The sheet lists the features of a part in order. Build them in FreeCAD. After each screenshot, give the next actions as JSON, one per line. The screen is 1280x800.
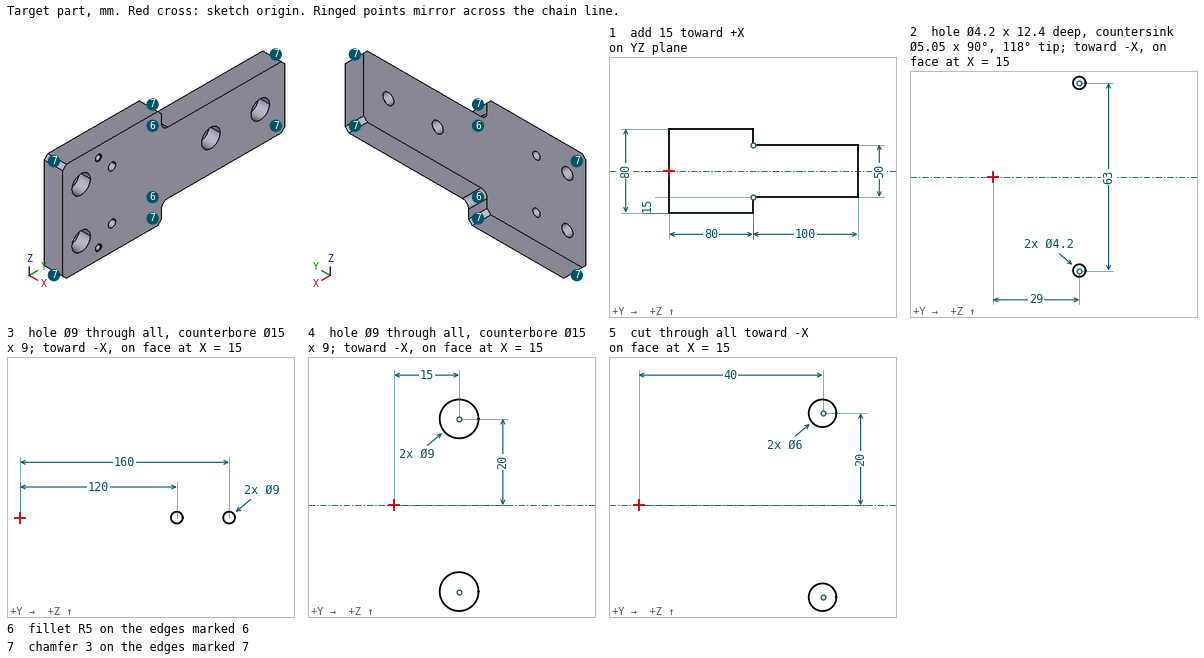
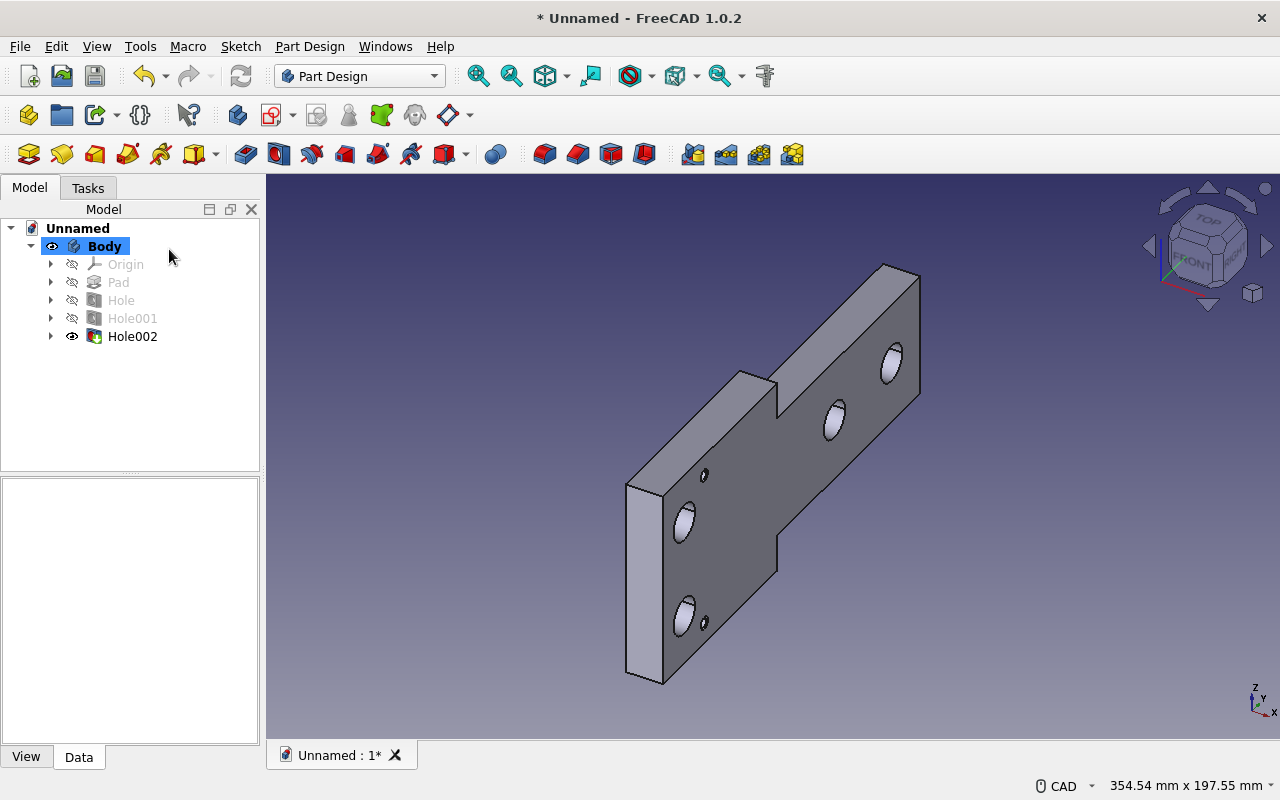
{"action": "left_click", "coordinate": [755, 498]}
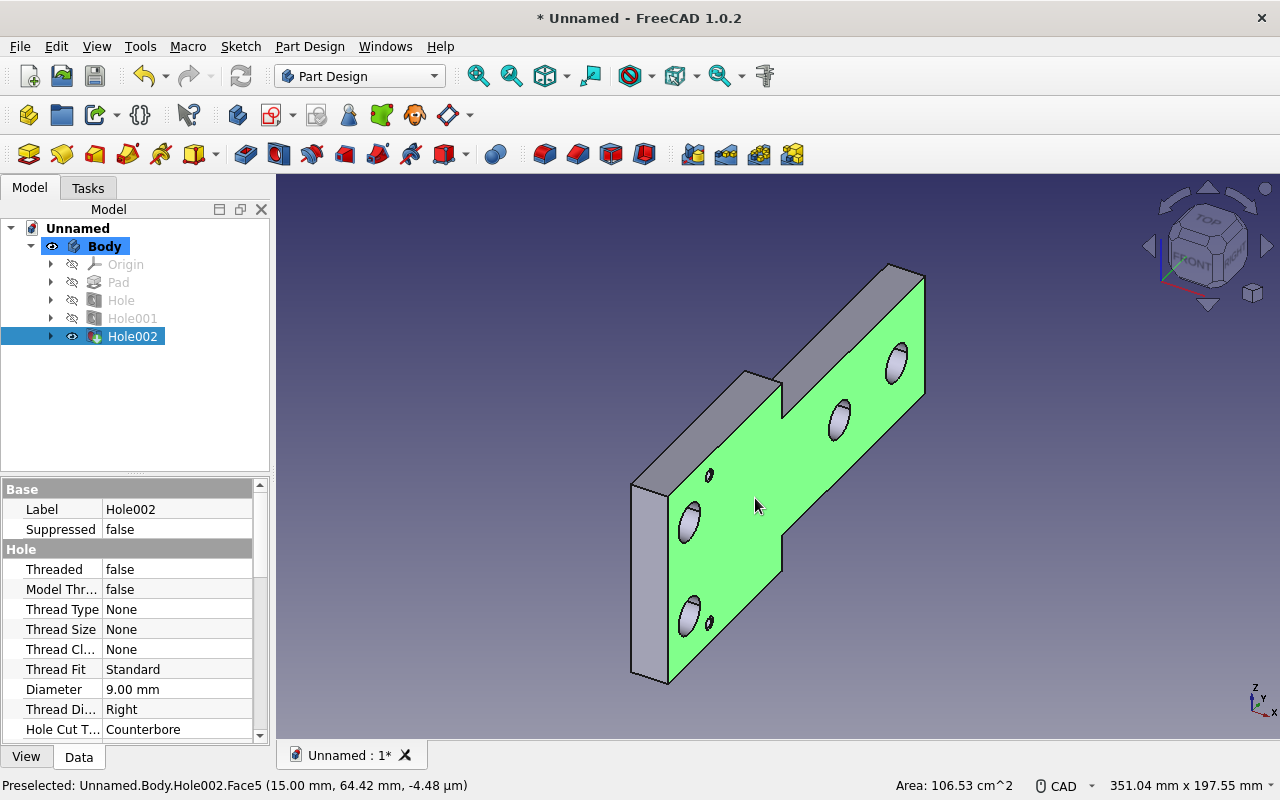
{"action": "left_click", "coordinate": [270, 116]}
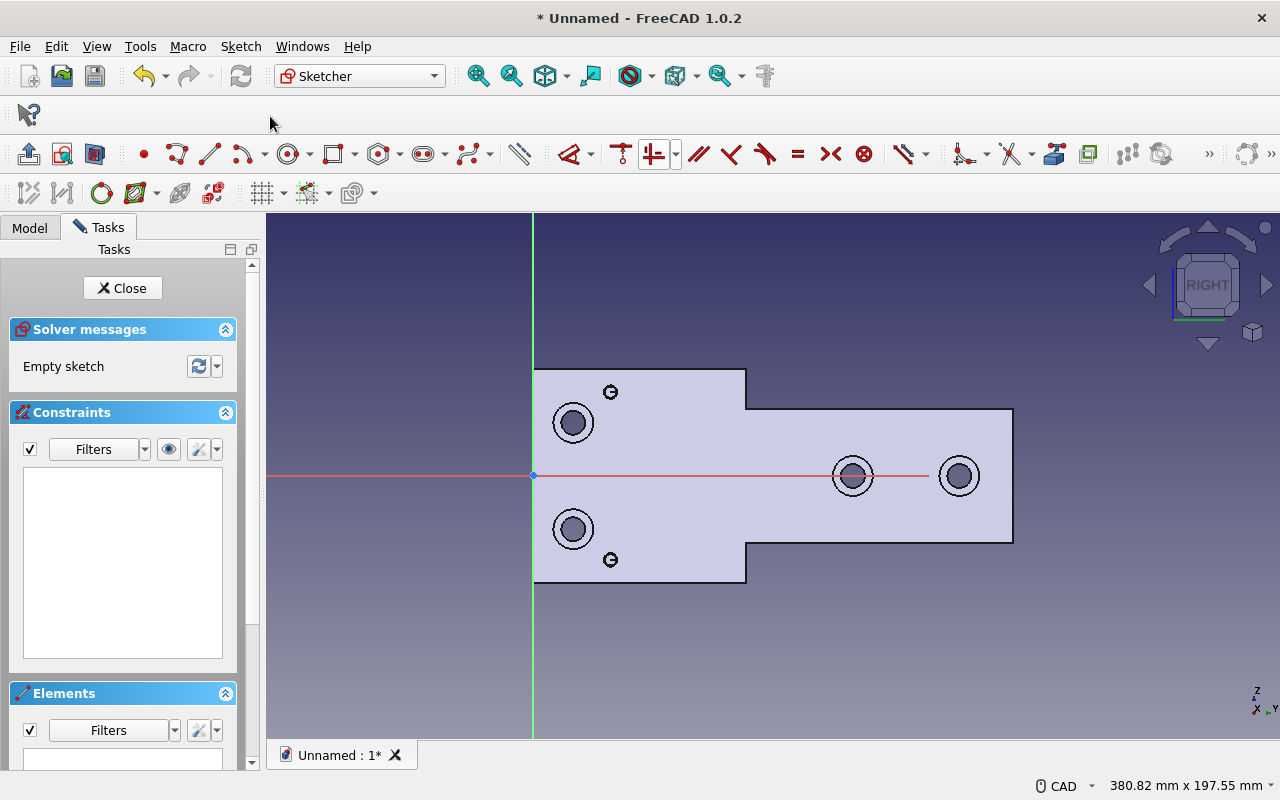
{"action": "scroll", "coordinate": [524, 476], "scroll_direction": "up", "scroll_amount": 5}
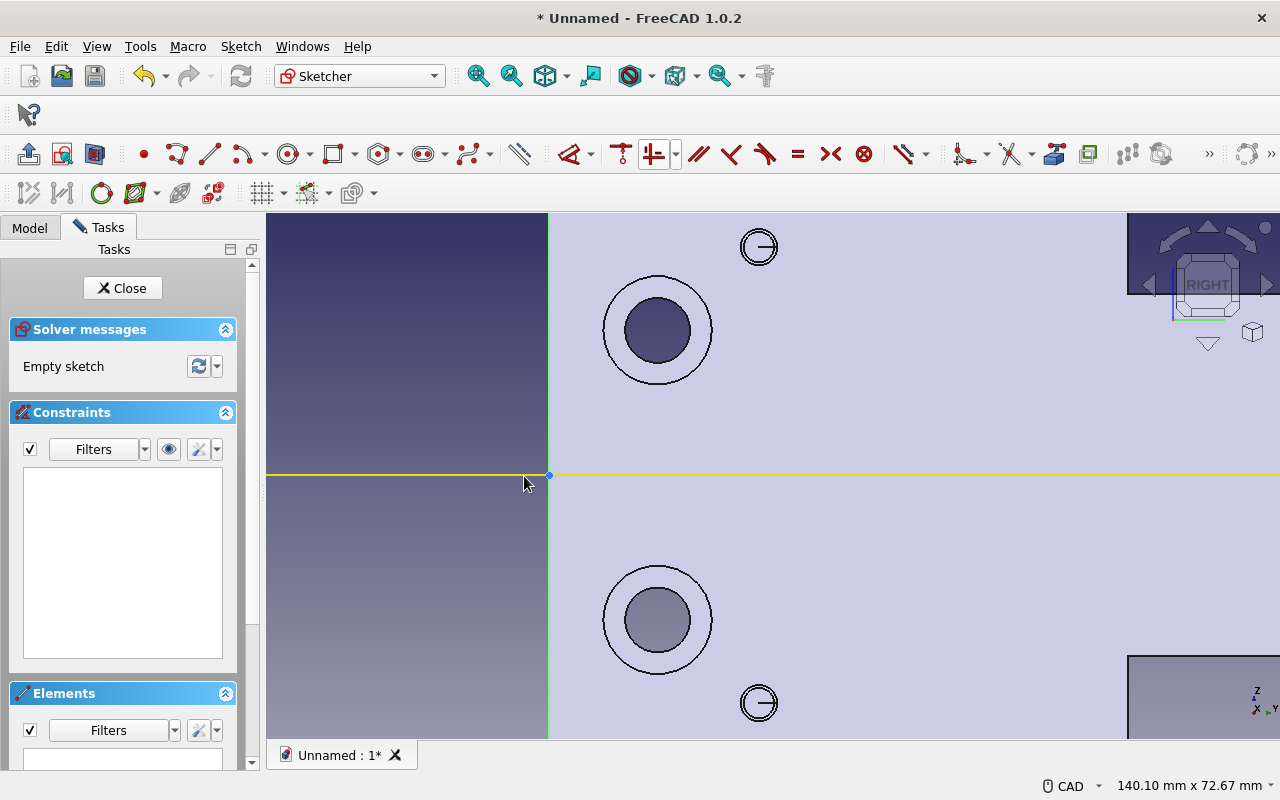
{"action": "left_click", "coordinate": [288, 154]}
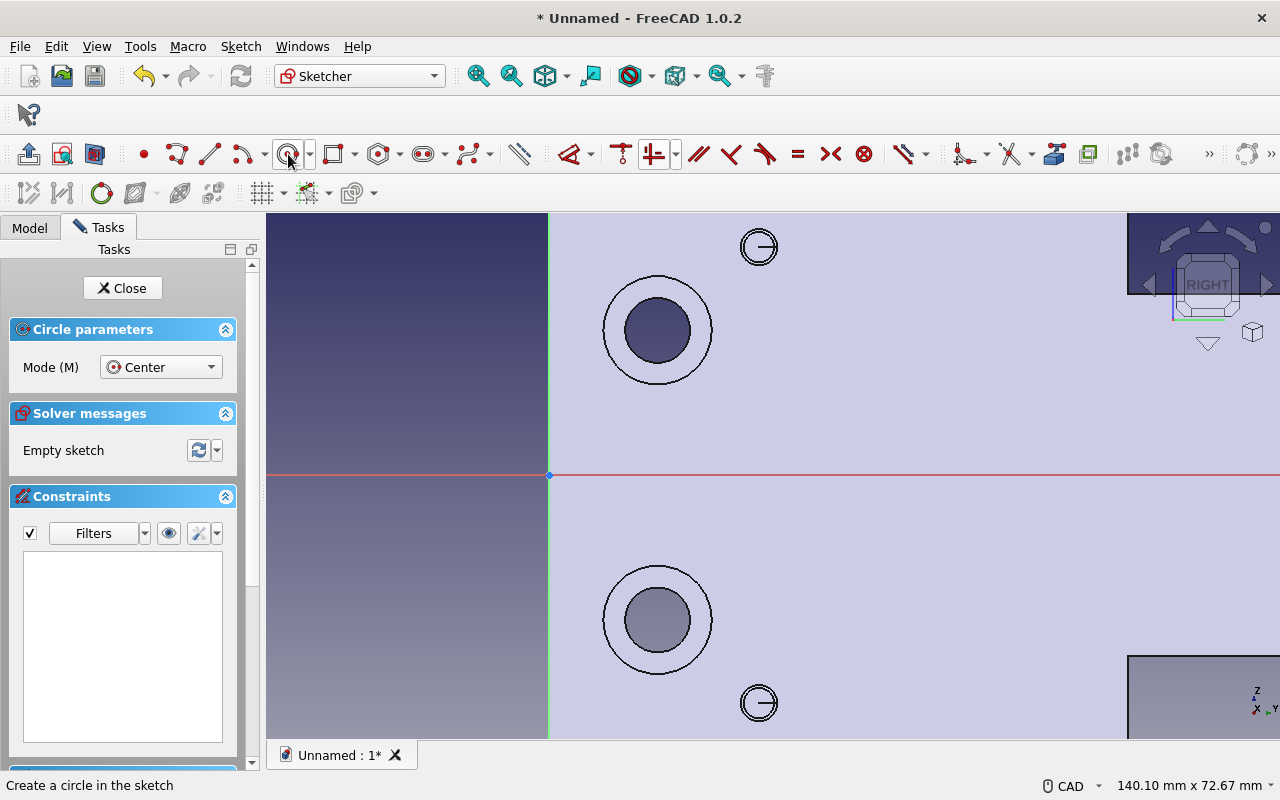
{"action": "left_click", "coordinate": [839, 330]}
{"action": "mouse_move", "coordinate": [854, 315]}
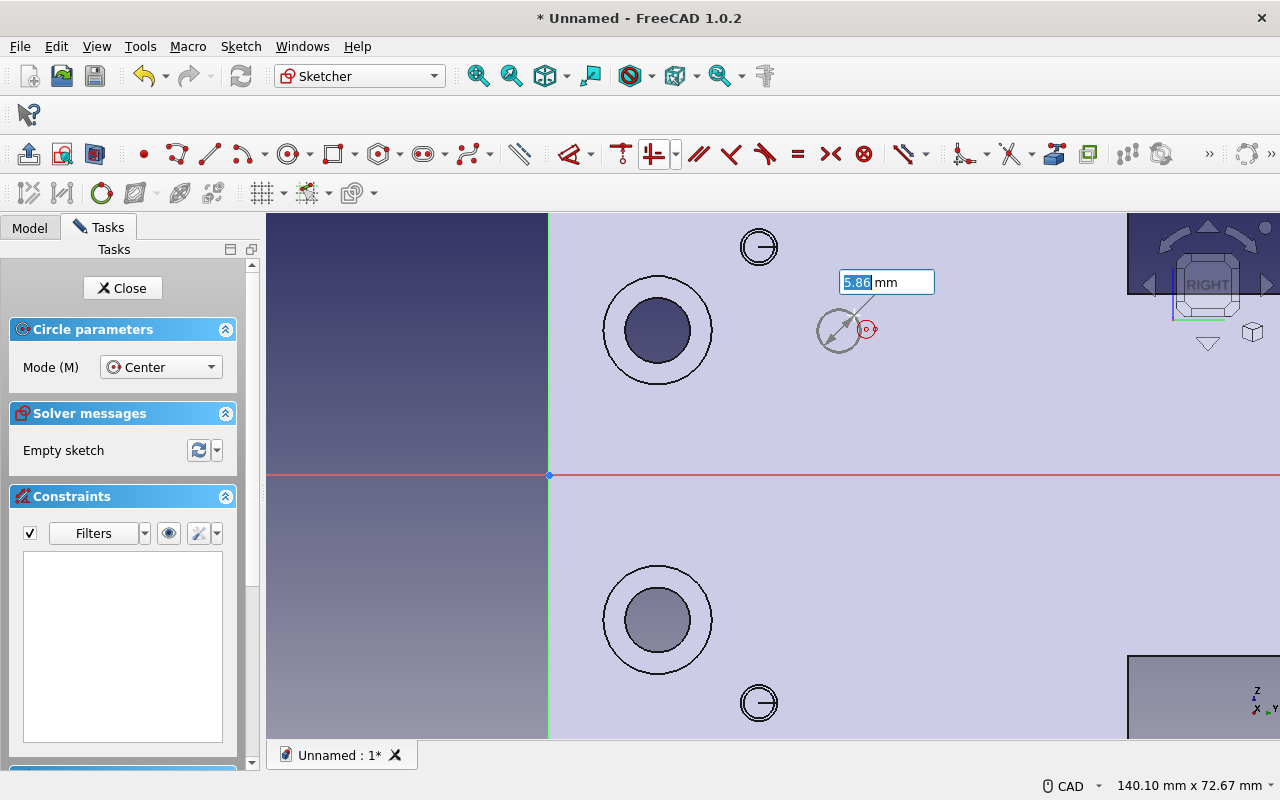
{"action": "type", "text": "6"}
{"action": "key", "text": "Return"}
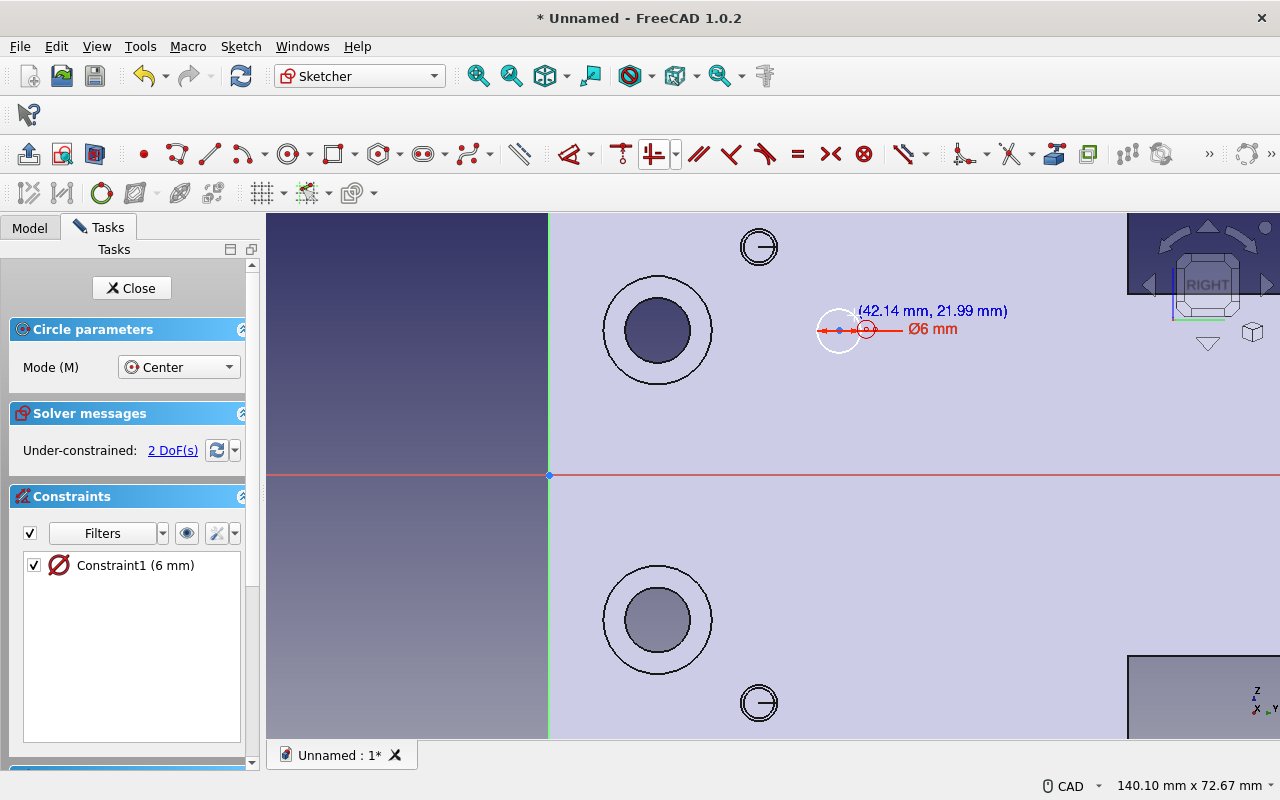
{"action": "left_click", "coordinate": [839, 620]}
{"action": "mouse_move", "coordinate": [854, 605]}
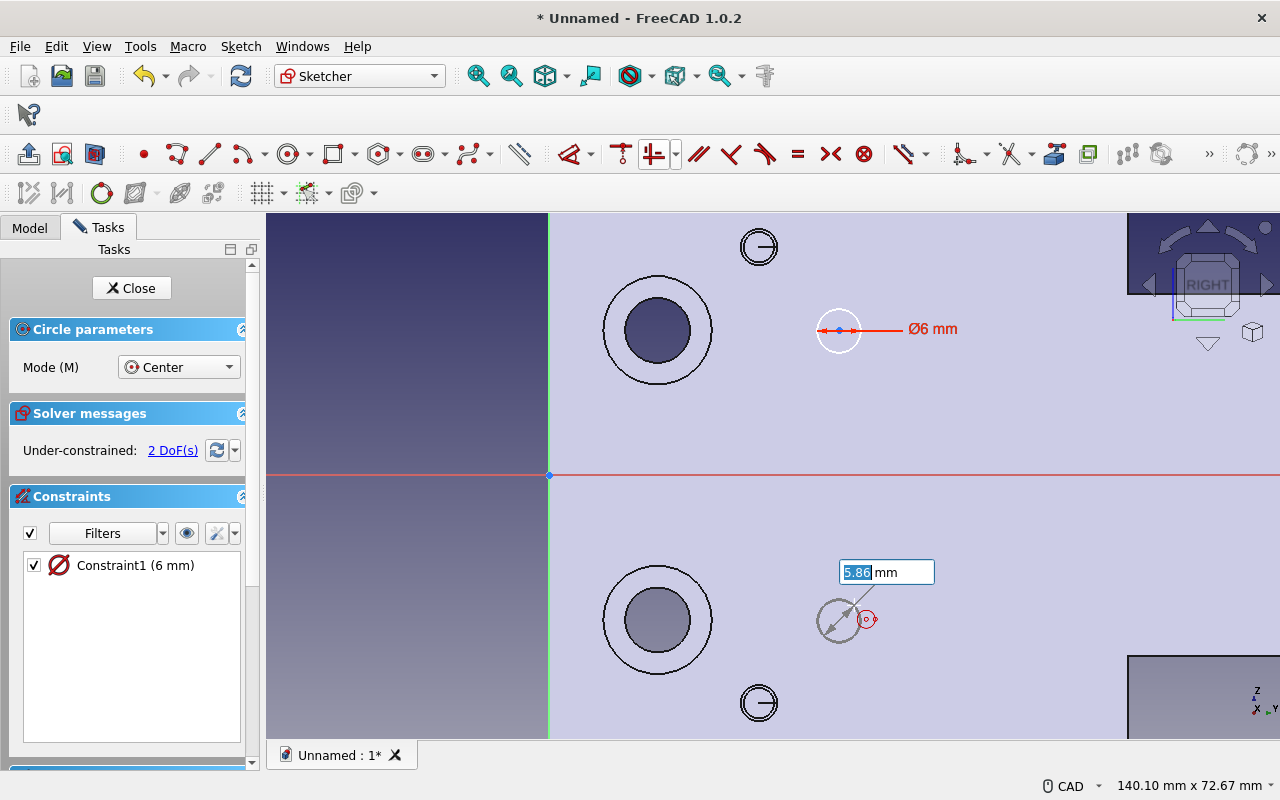
{"action": "type", "text": "6"}
{"action": "key", "text": "Return"}
{"action": "key", "text": "Escape"}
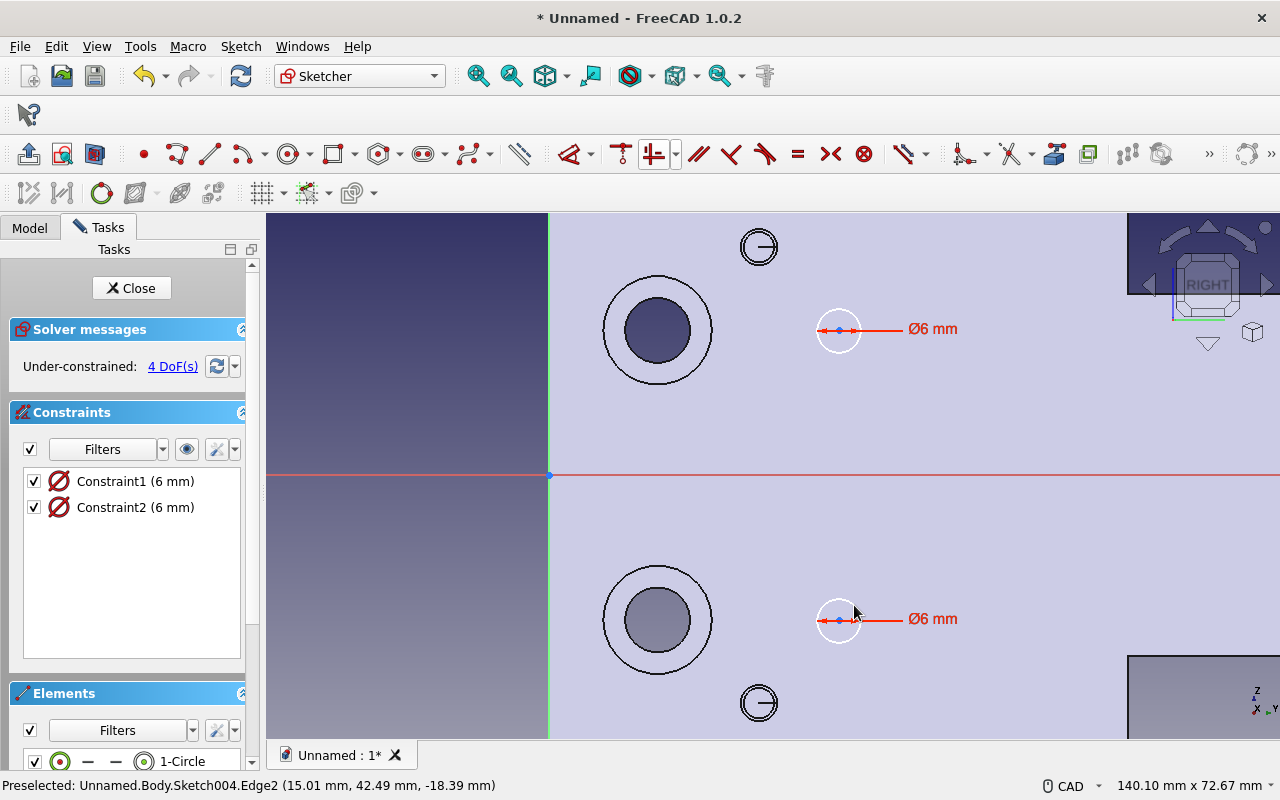
{"action": "left_click", "coordinate": [839, 331]}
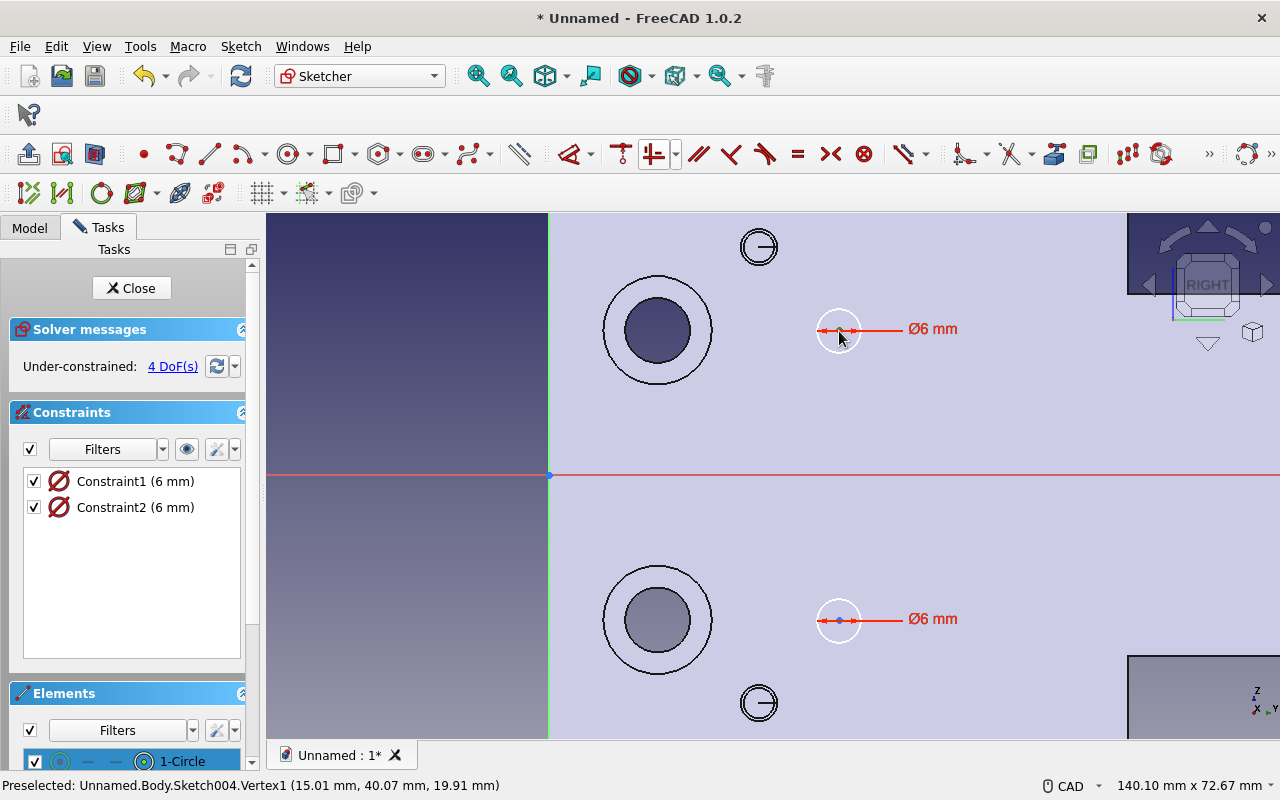
{"action": "left_click", "coordinate": [839, 621]}